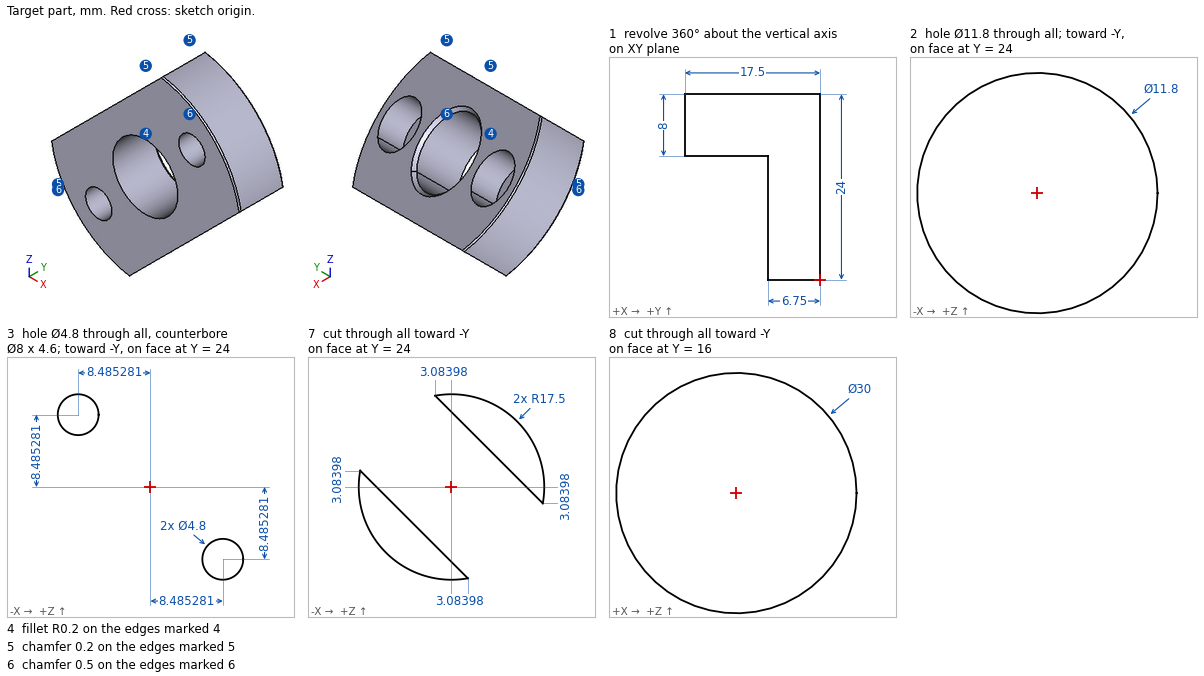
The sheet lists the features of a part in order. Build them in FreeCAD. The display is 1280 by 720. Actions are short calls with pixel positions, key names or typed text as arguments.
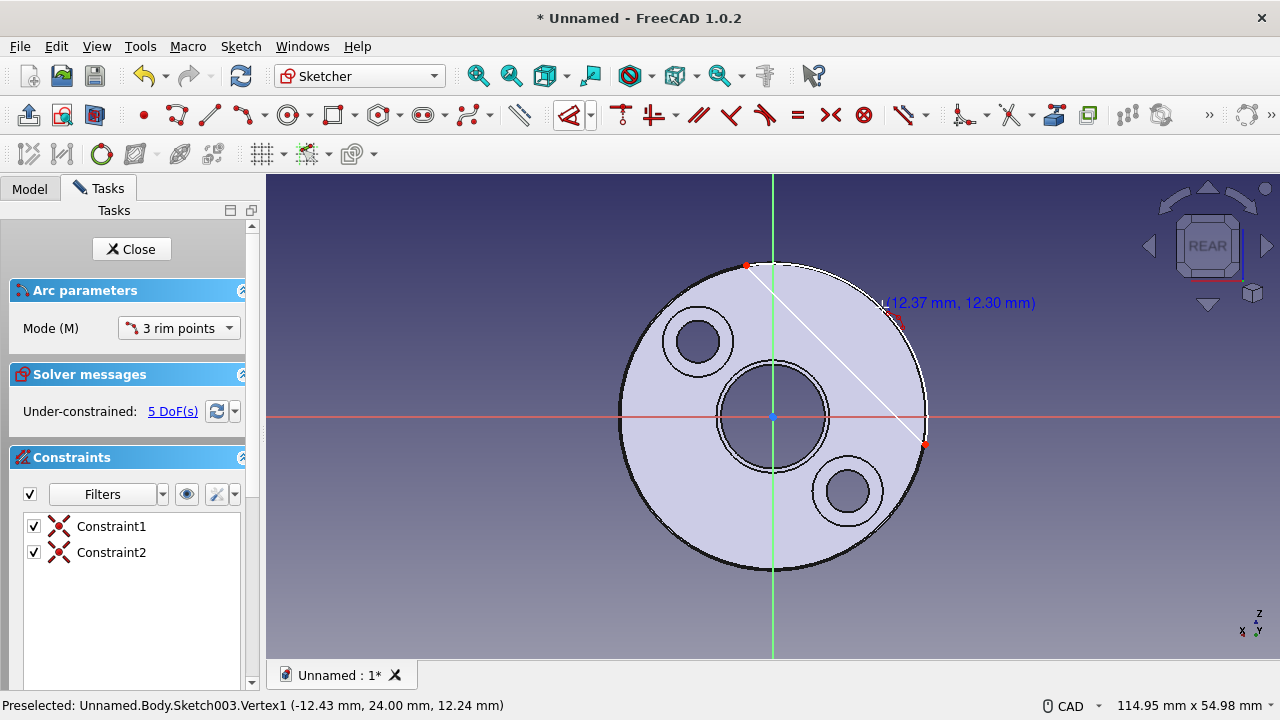
click(210, 116)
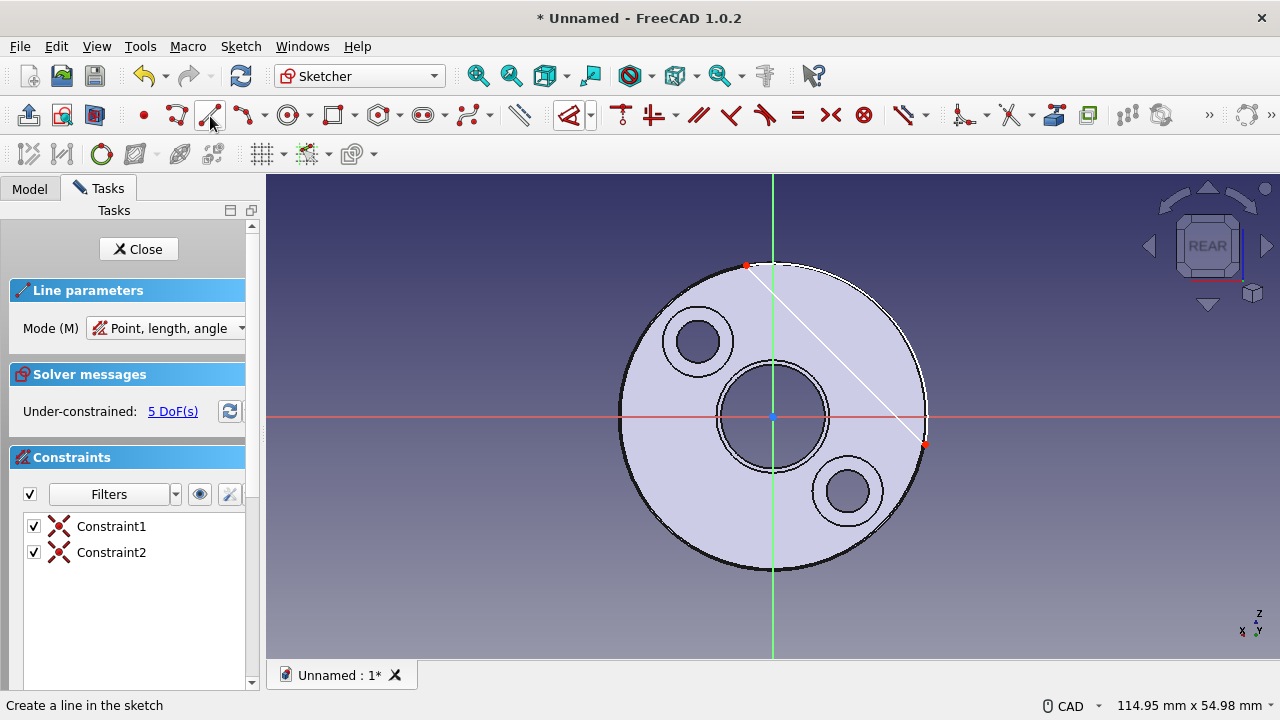
click(800, 568)
click(621, 389)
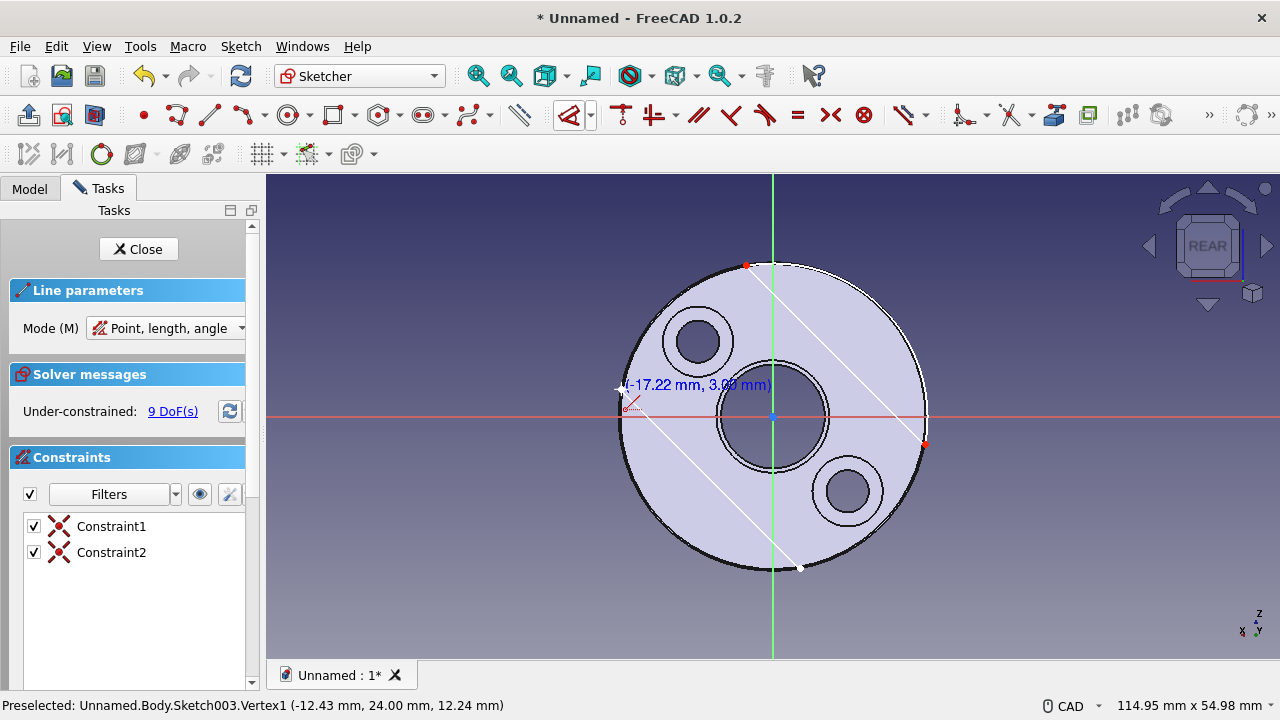
key(g)
key(3)
key(a)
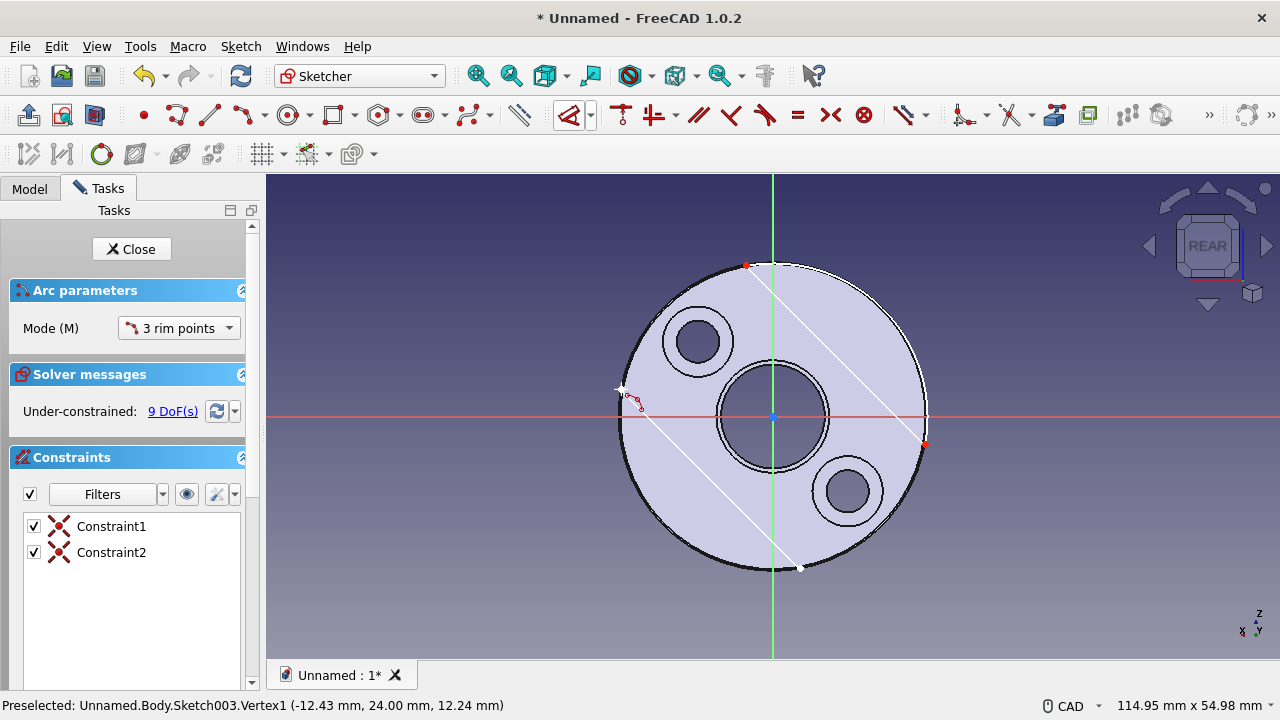
click(621, 390)
click(800, 569)
click(664, 526)
key(Escape)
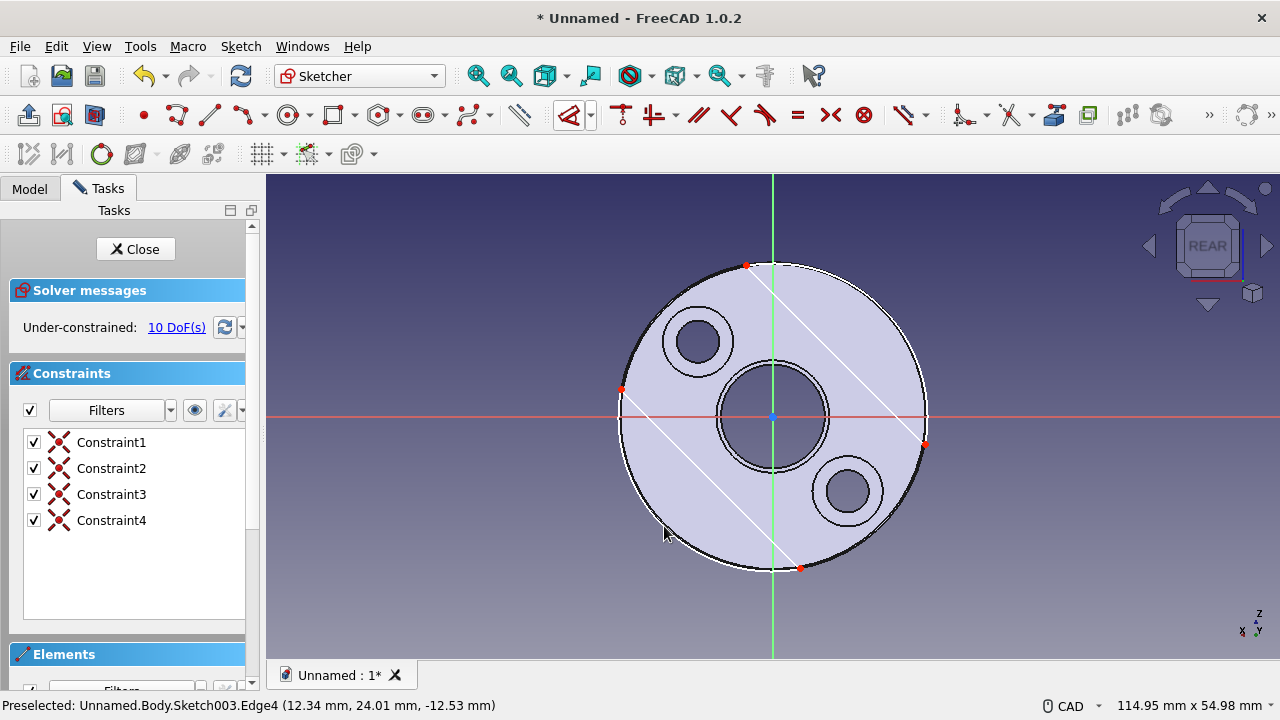
click(915, 358)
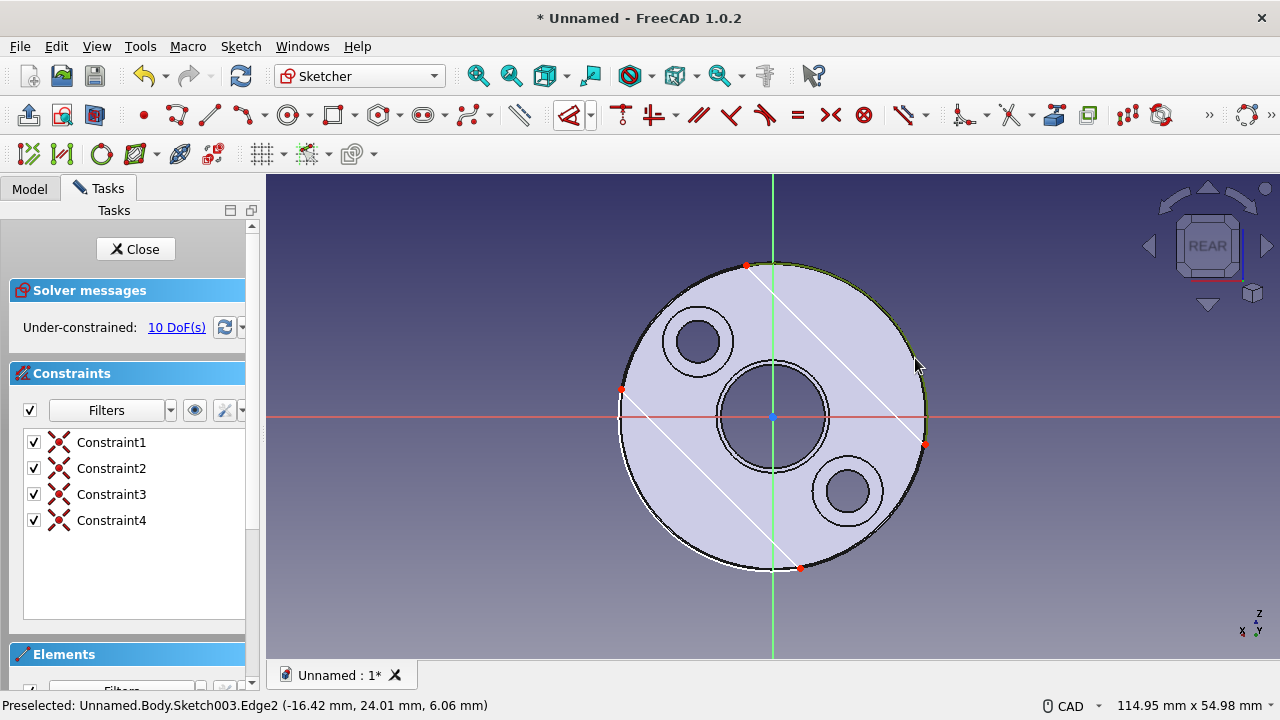
click(631, 477)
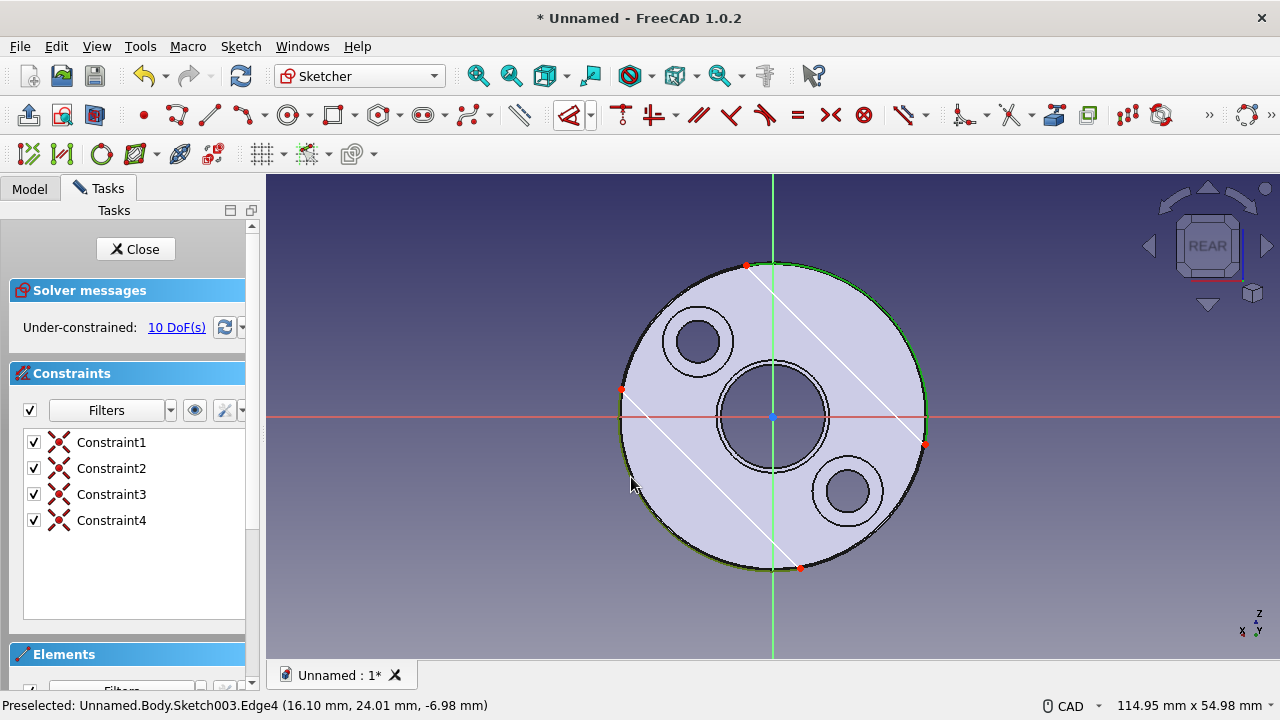
click(621, 116)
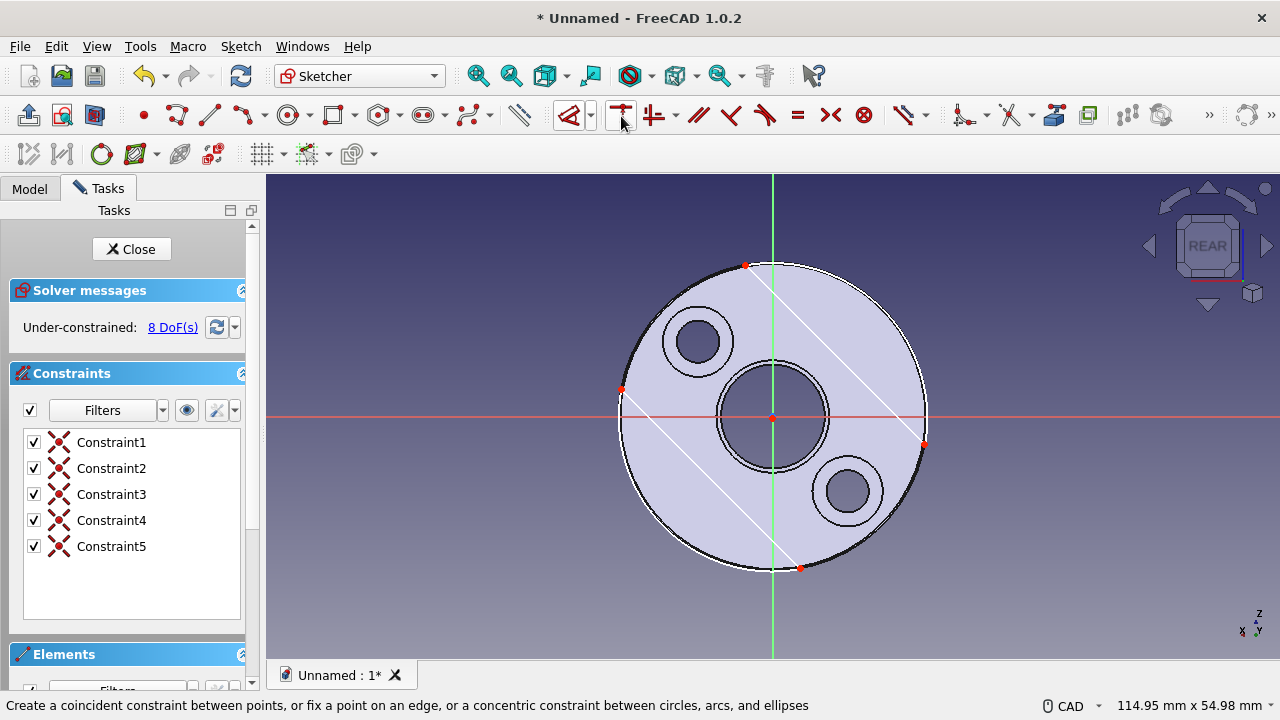
drag(762, 406, 783, 428)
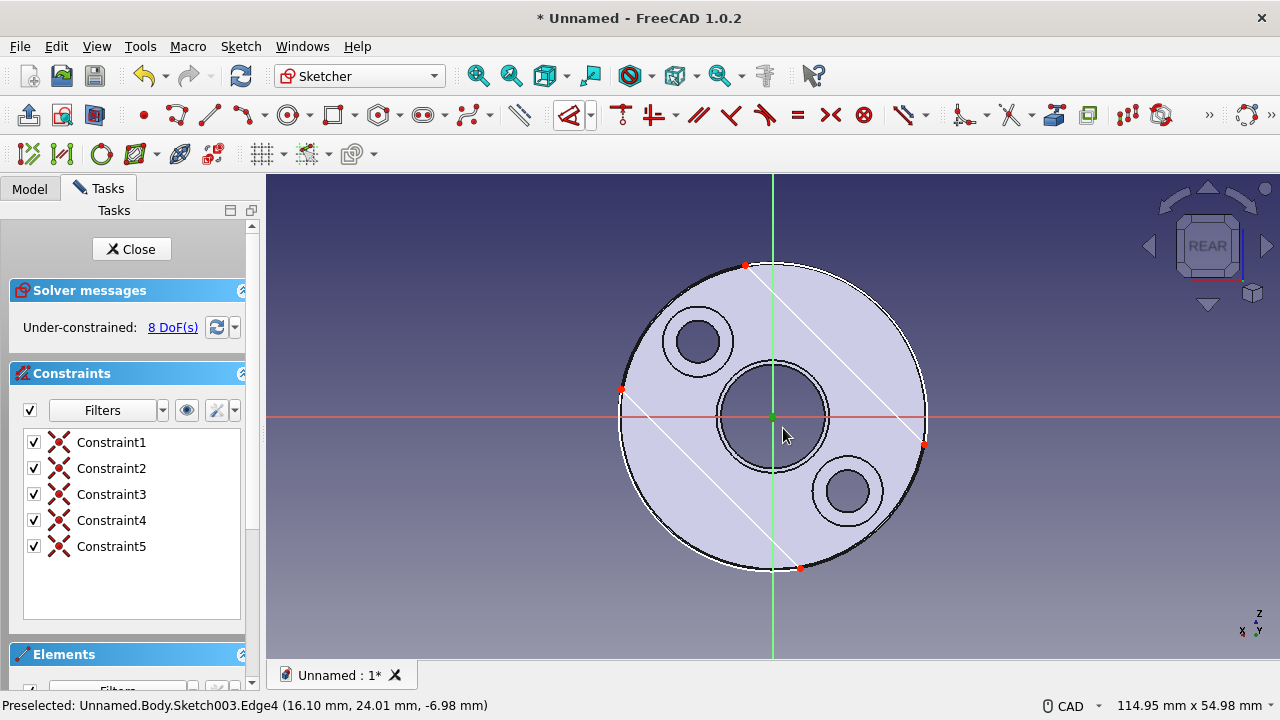
click(621, 116)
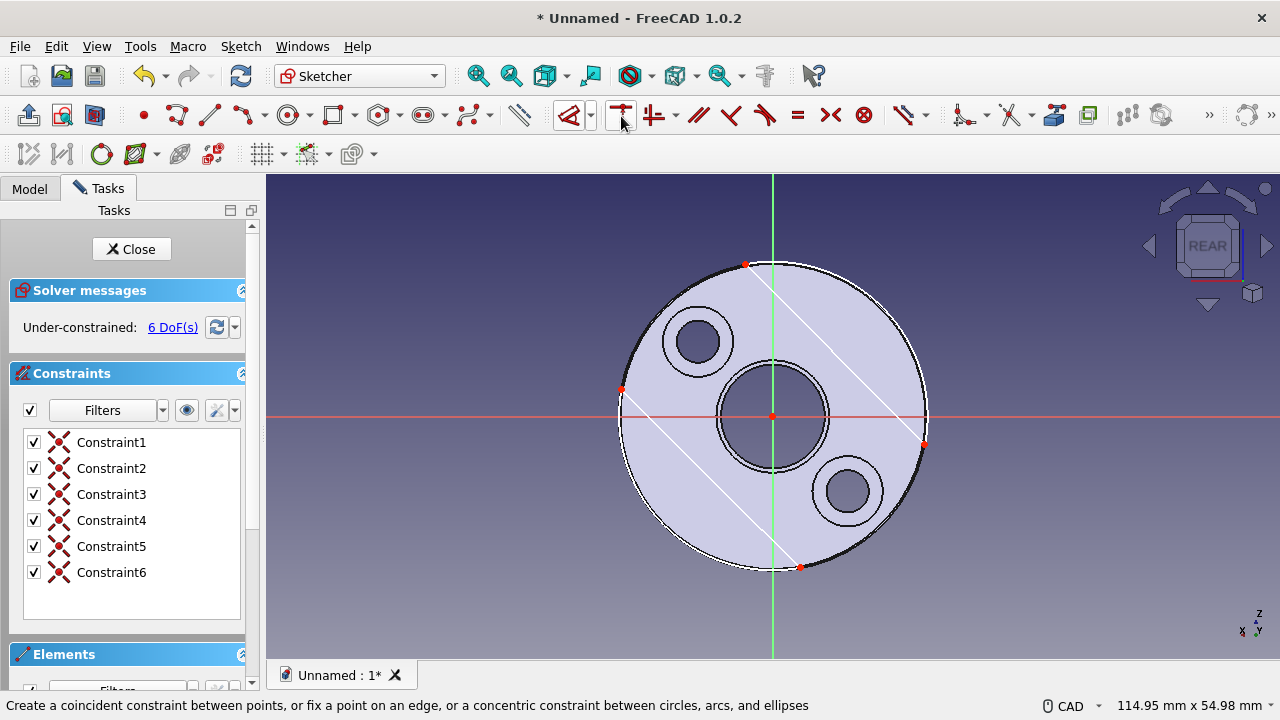
click(916, 357)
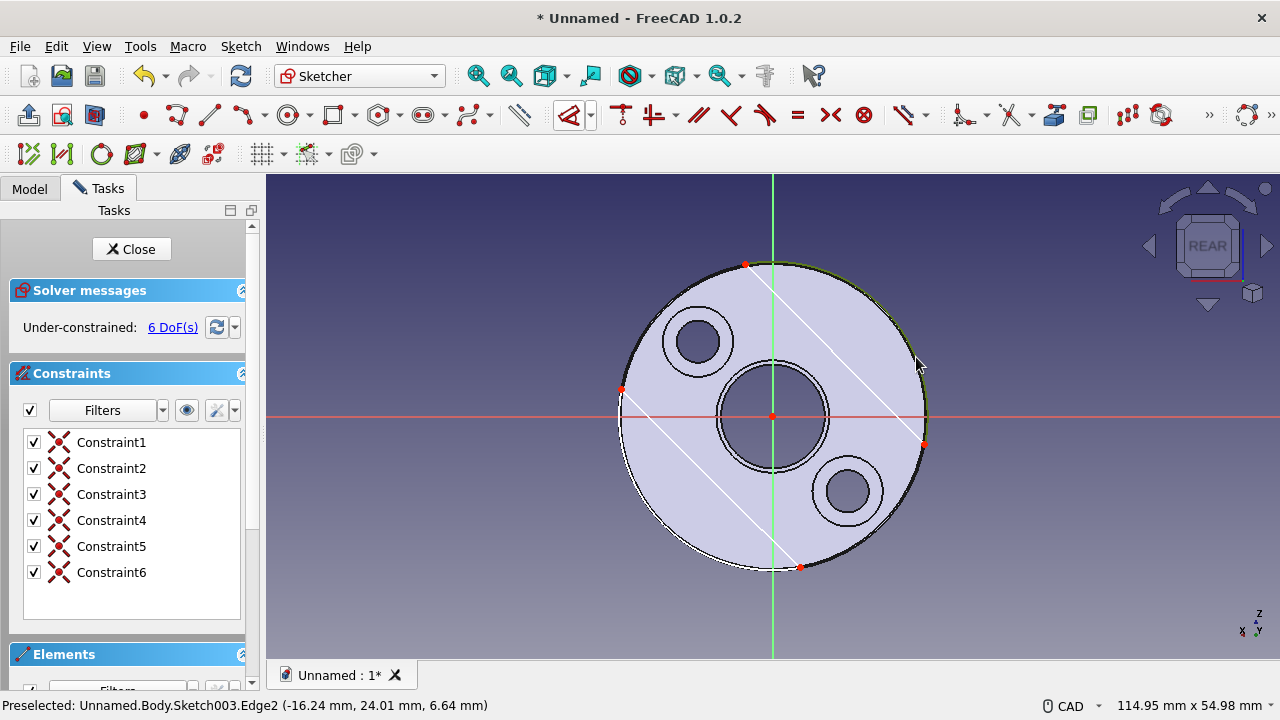
click(631, 477)